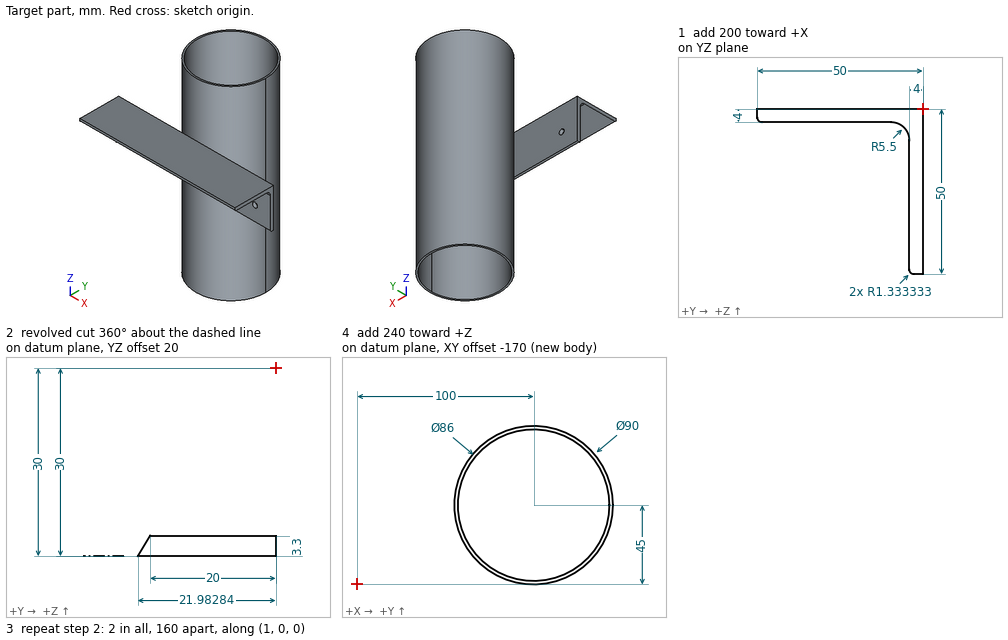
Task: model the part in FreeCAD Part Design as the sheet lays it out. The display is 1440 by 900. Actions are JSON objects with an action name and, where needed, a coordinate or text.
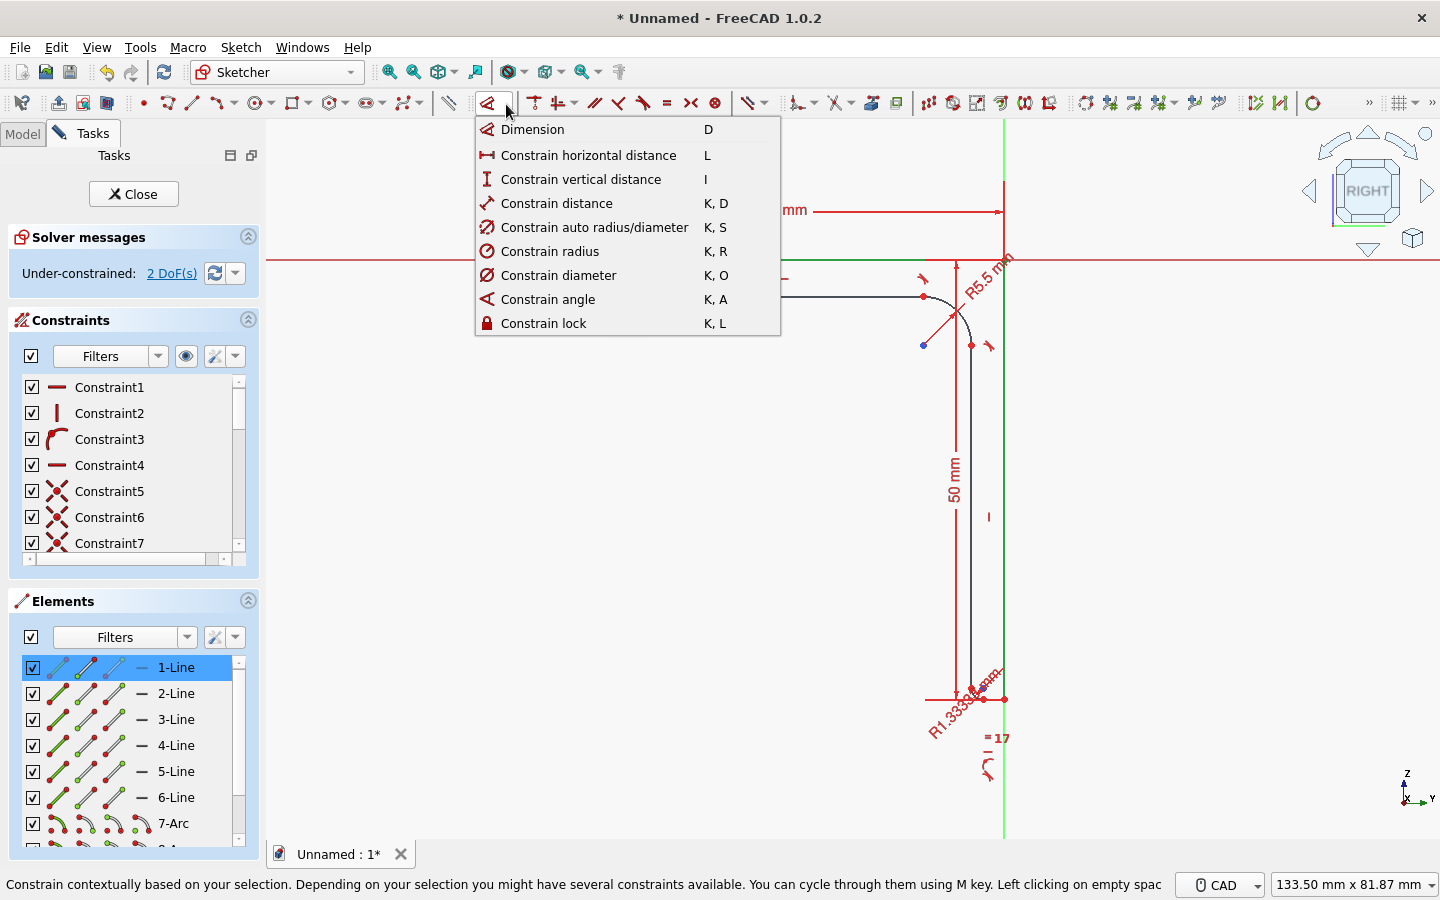
{"action": "left_click", "coordinate": [628, 179]}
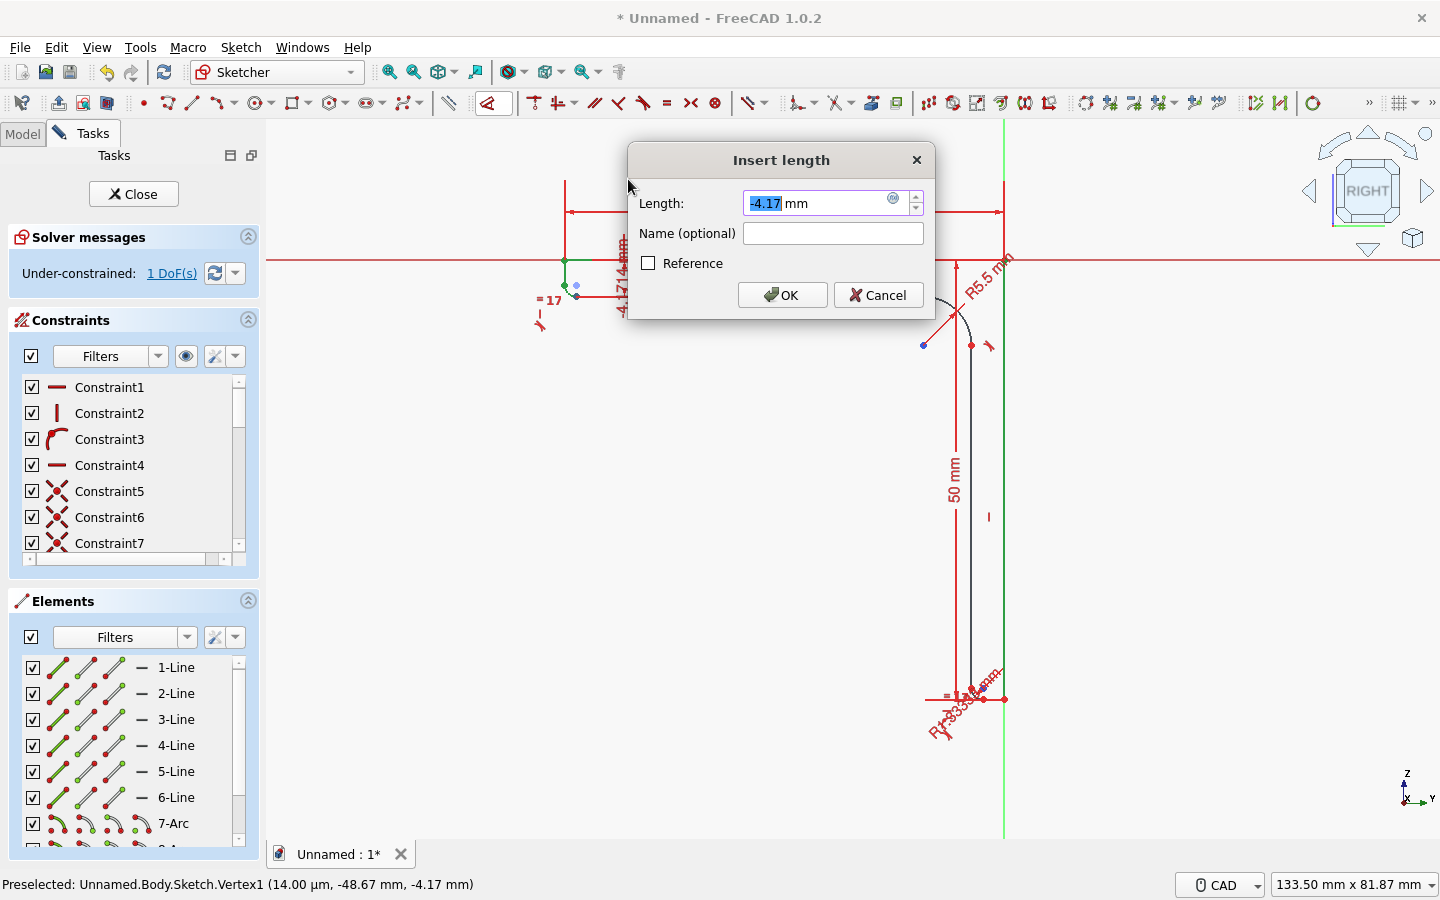
{"action": "type", "text": "-4"}
{"action": "key", "text": "Return"}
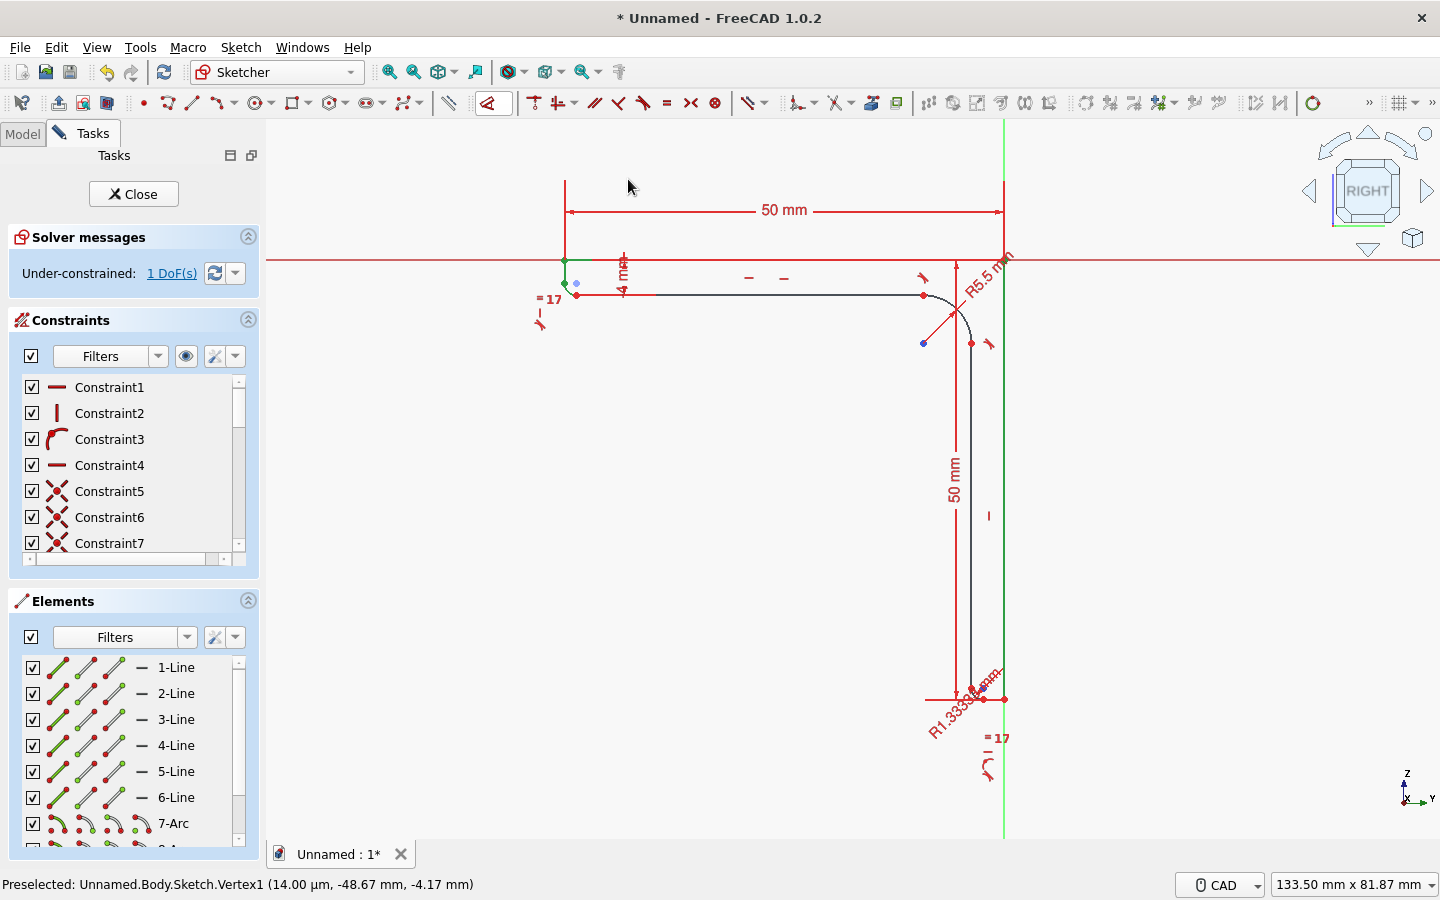
{"action": "left_click", "coordinate": [971, 344]}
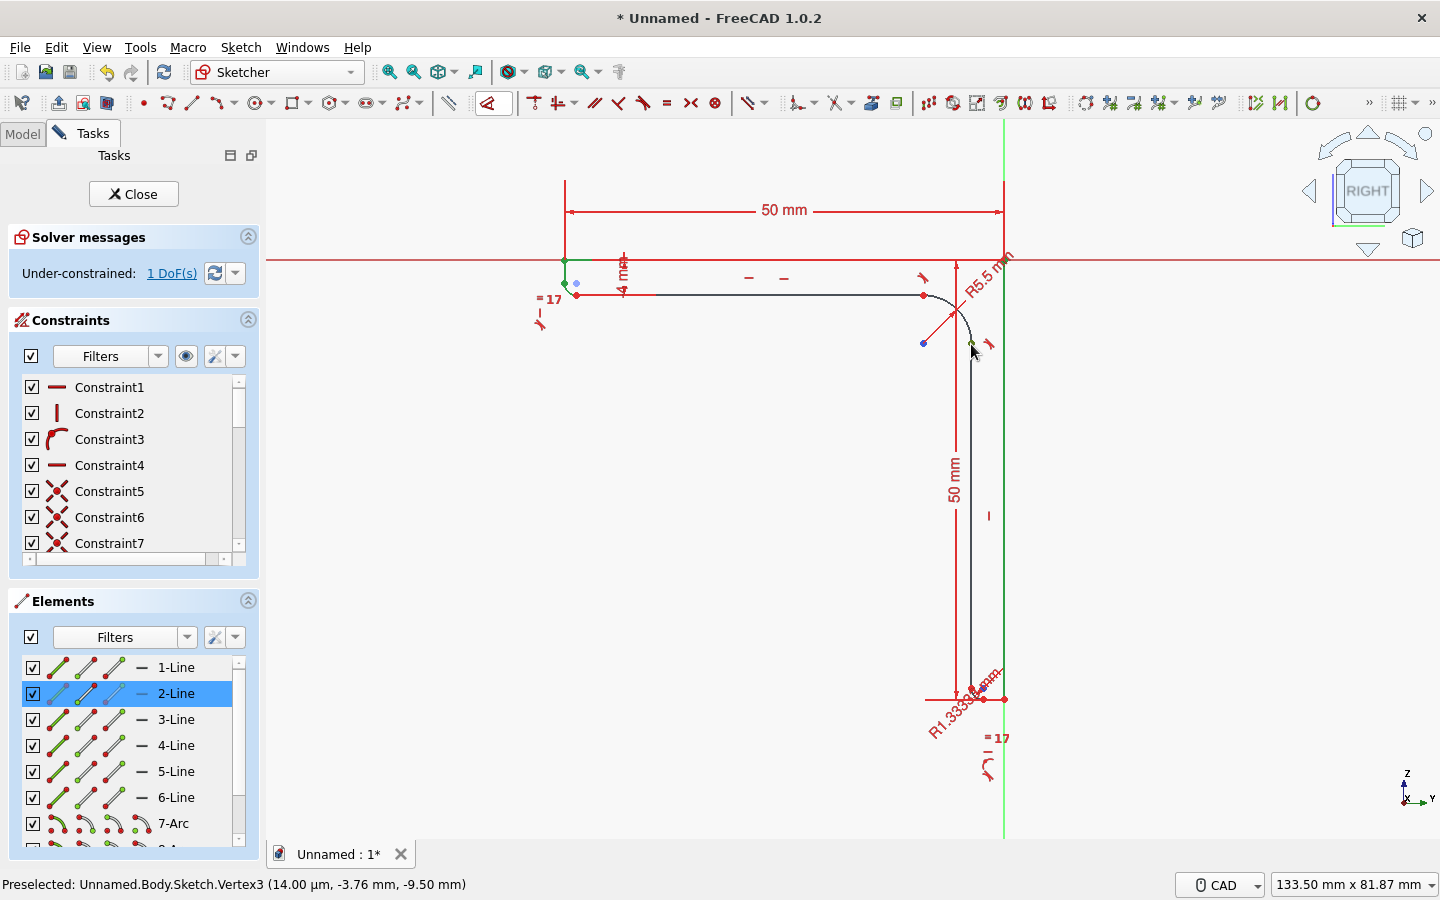
{"action": "left_click", "coordinate": [506, 104]}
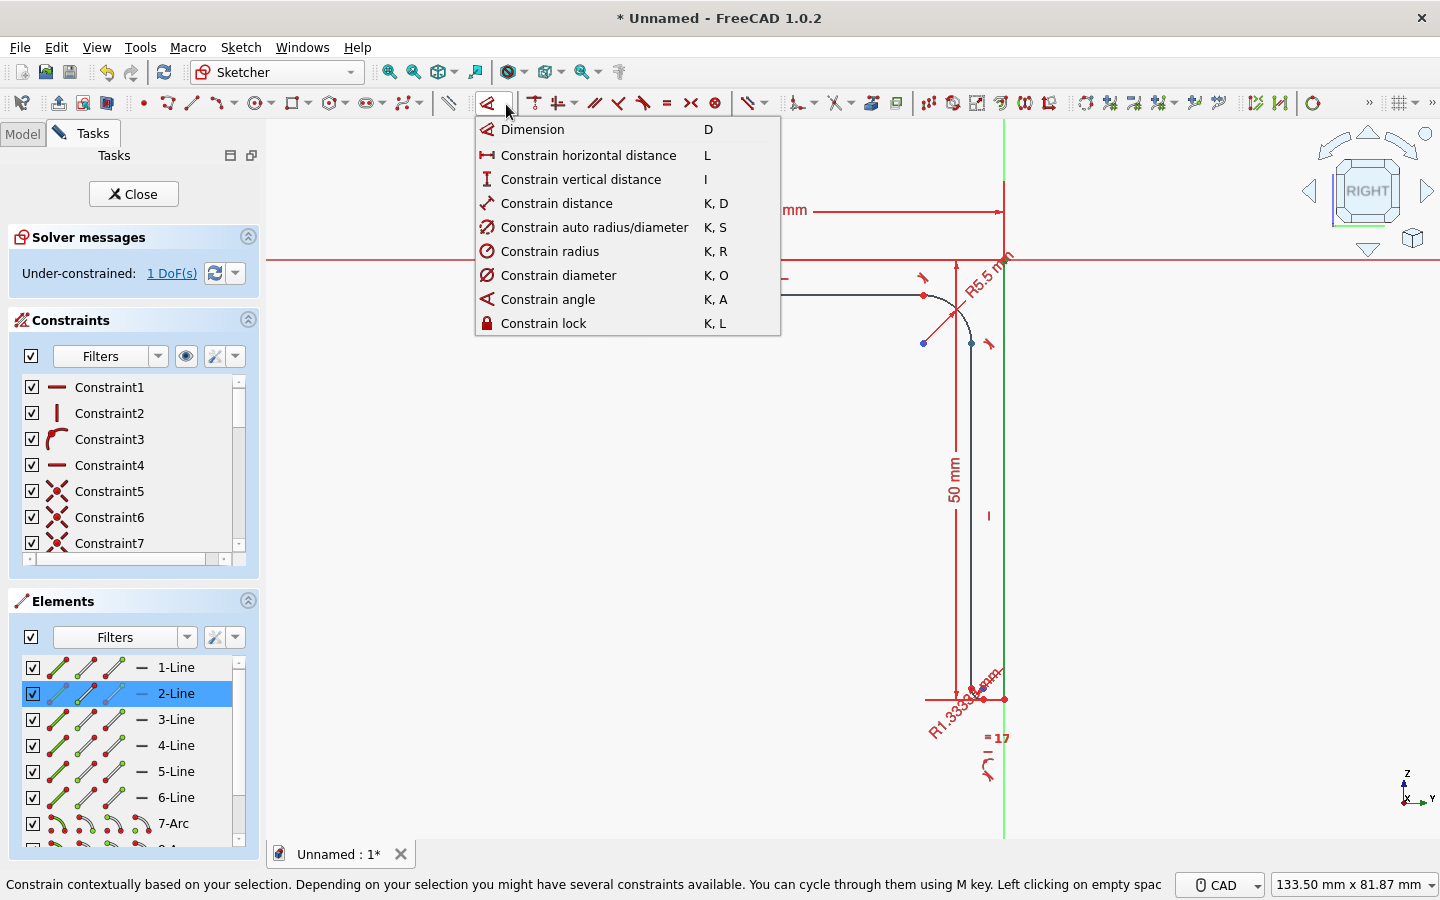
{"action": "left_click", "coordinate": [628, 155]}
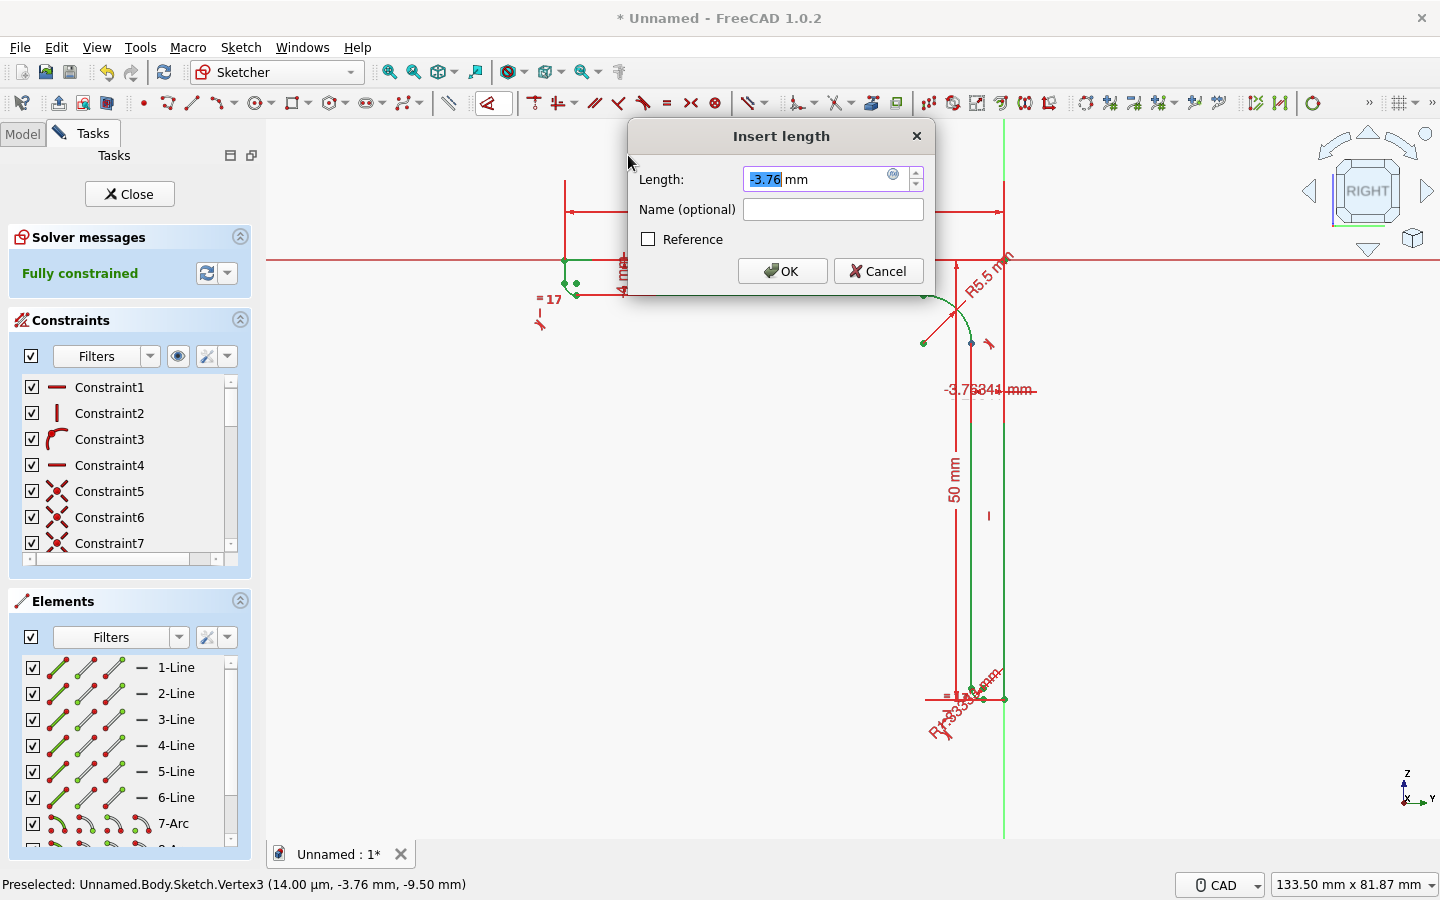
{"action": "type", "text": "-4"}
{"action": "key", "text": "Return"}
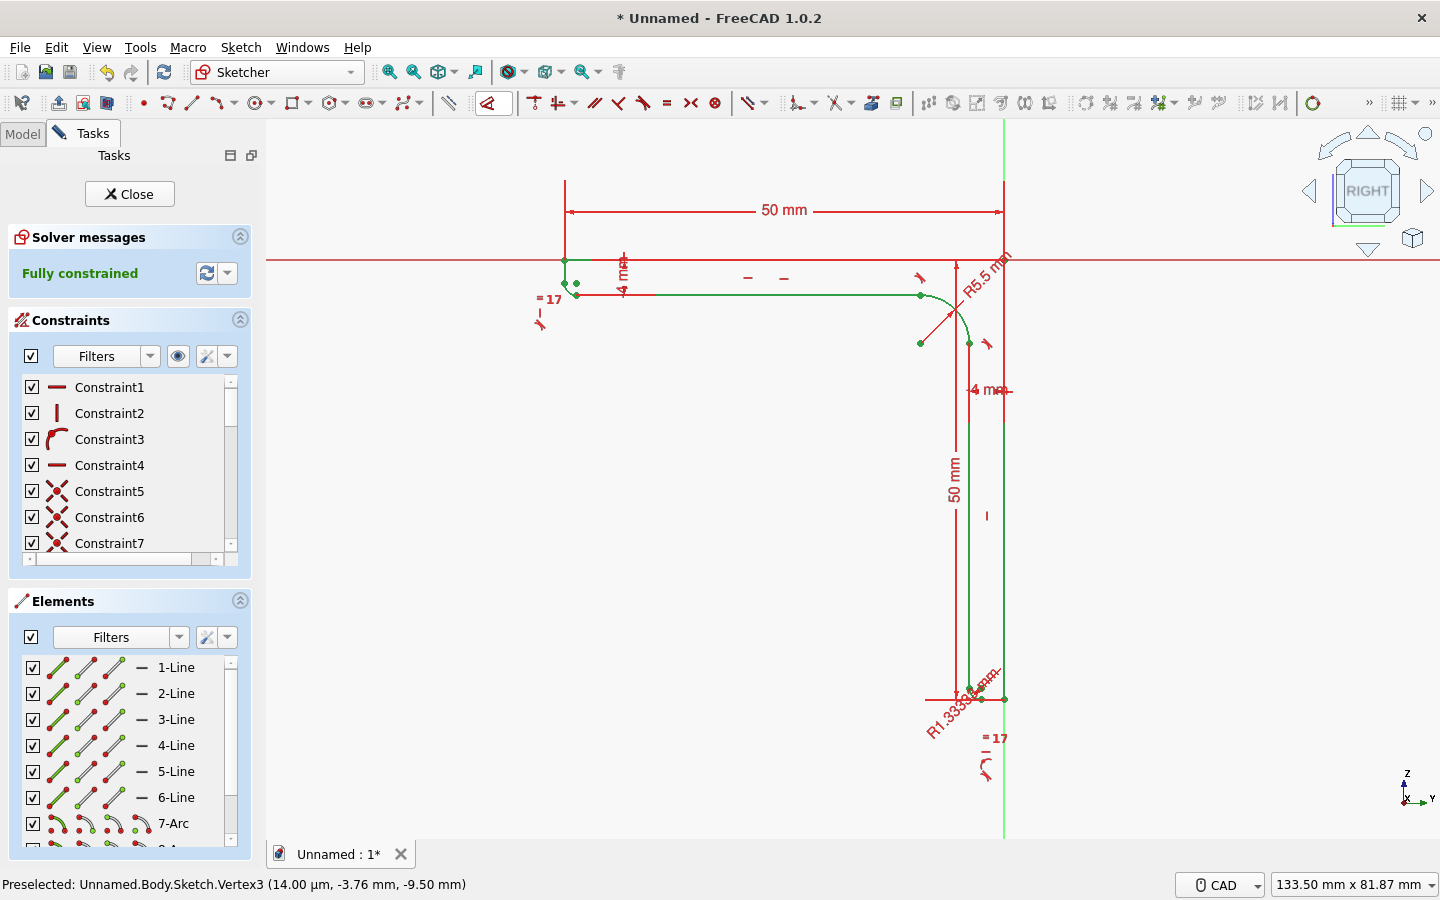
{"action": "left_click", "coordinate": [130, 194]}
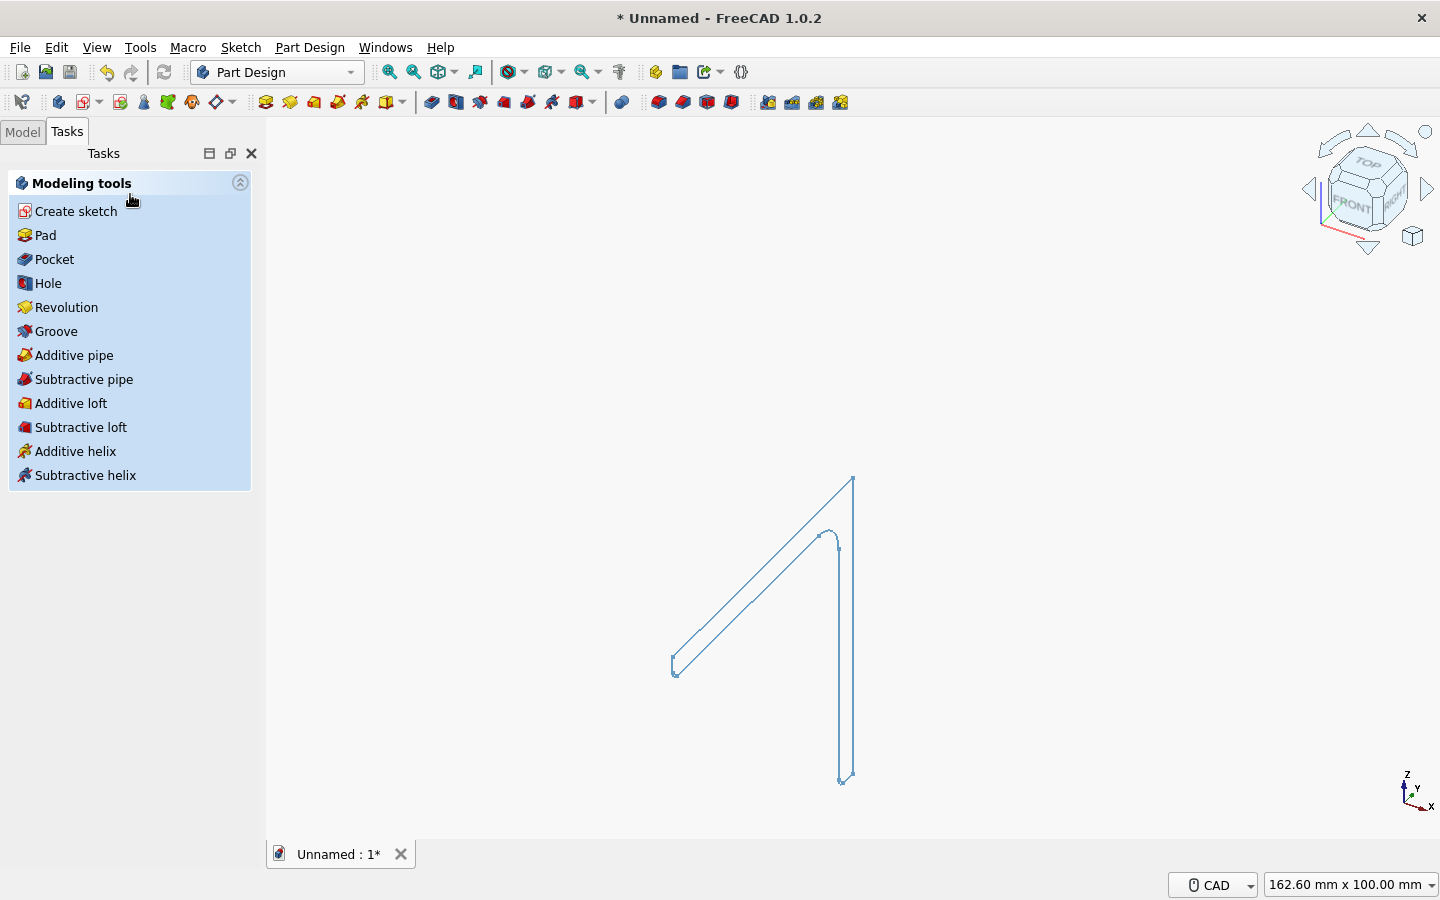
{"action": "left_click", "coordinate": [266, 102]}